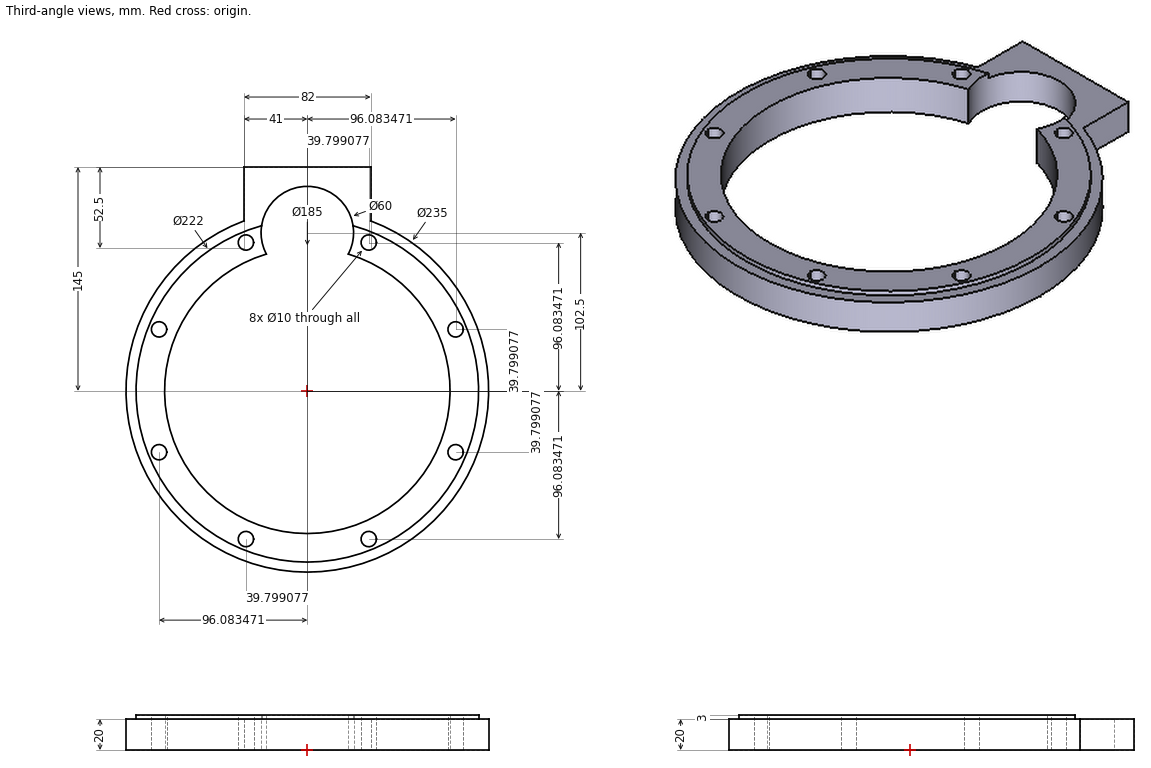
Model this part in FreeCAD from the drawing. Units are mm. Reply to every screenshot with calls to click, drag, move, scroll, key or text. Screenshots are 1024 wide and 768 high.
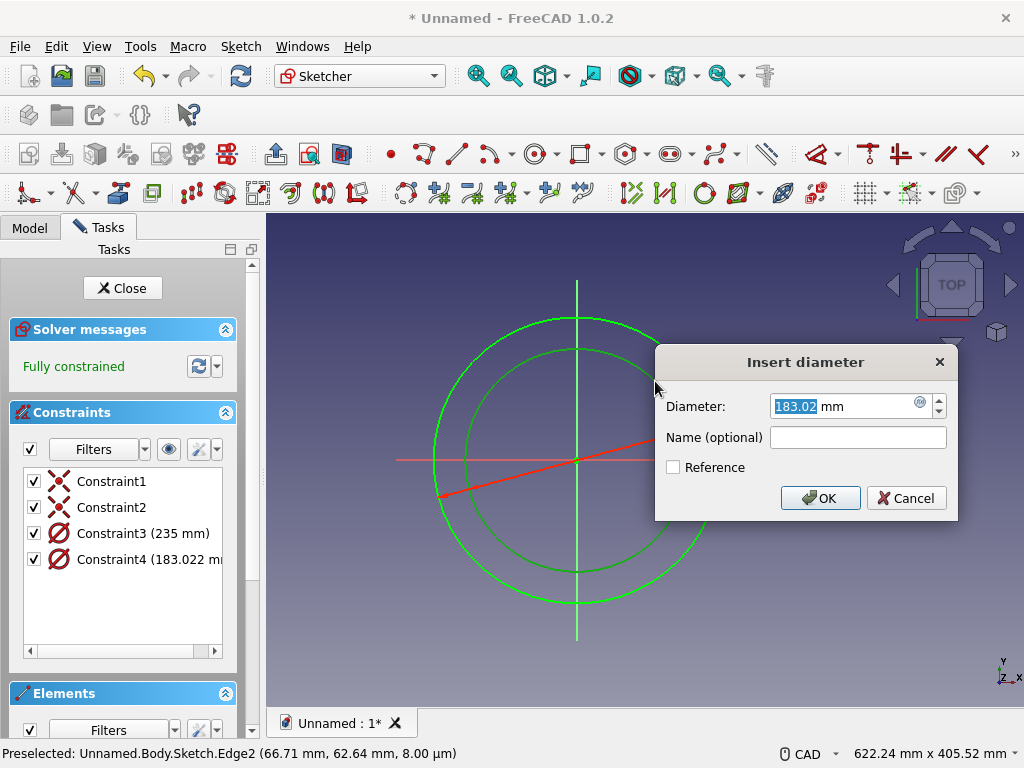
text(185)
key(Return)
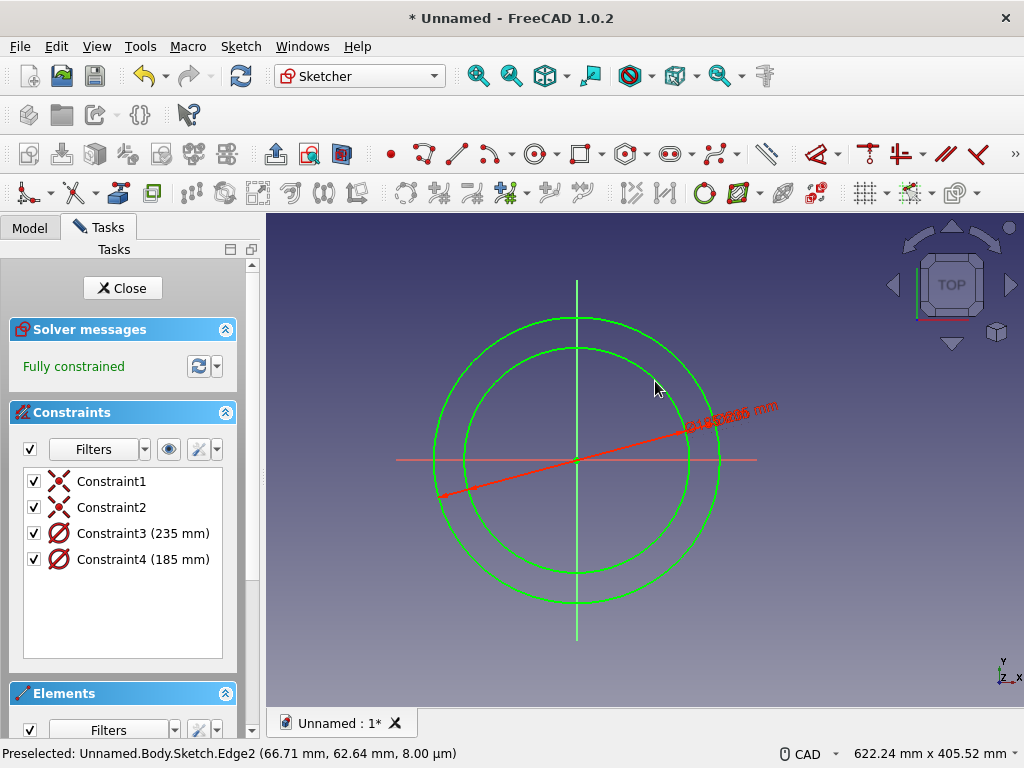
click(123, 288)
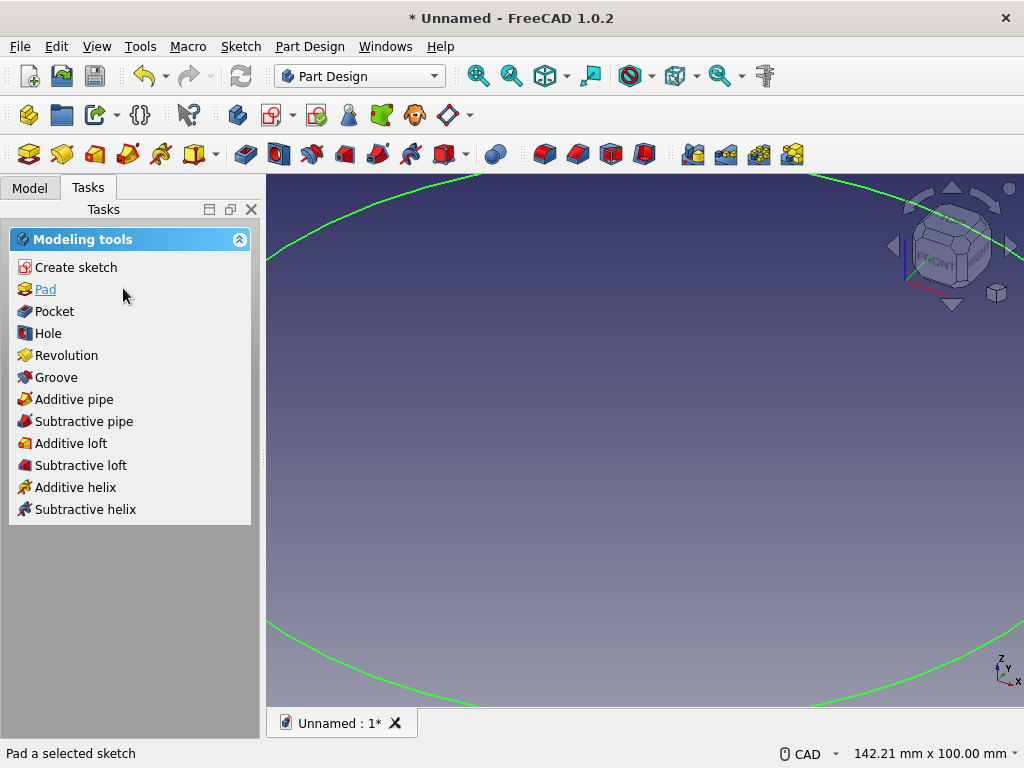
click(29, 154)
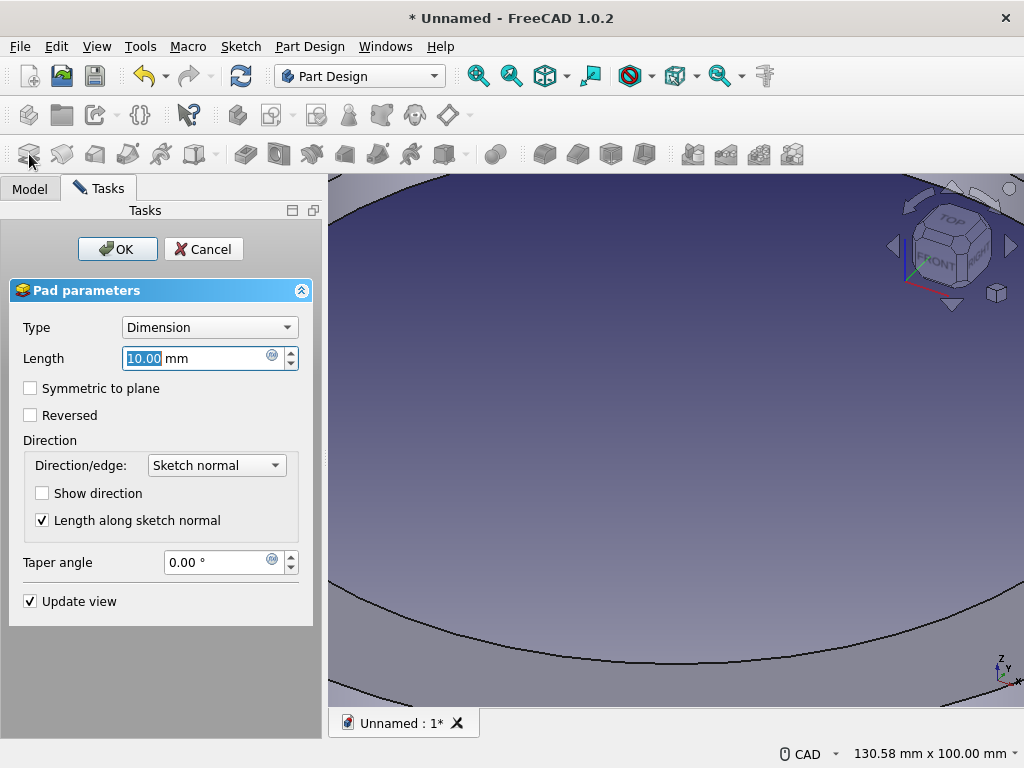
text(20)
key(Tab)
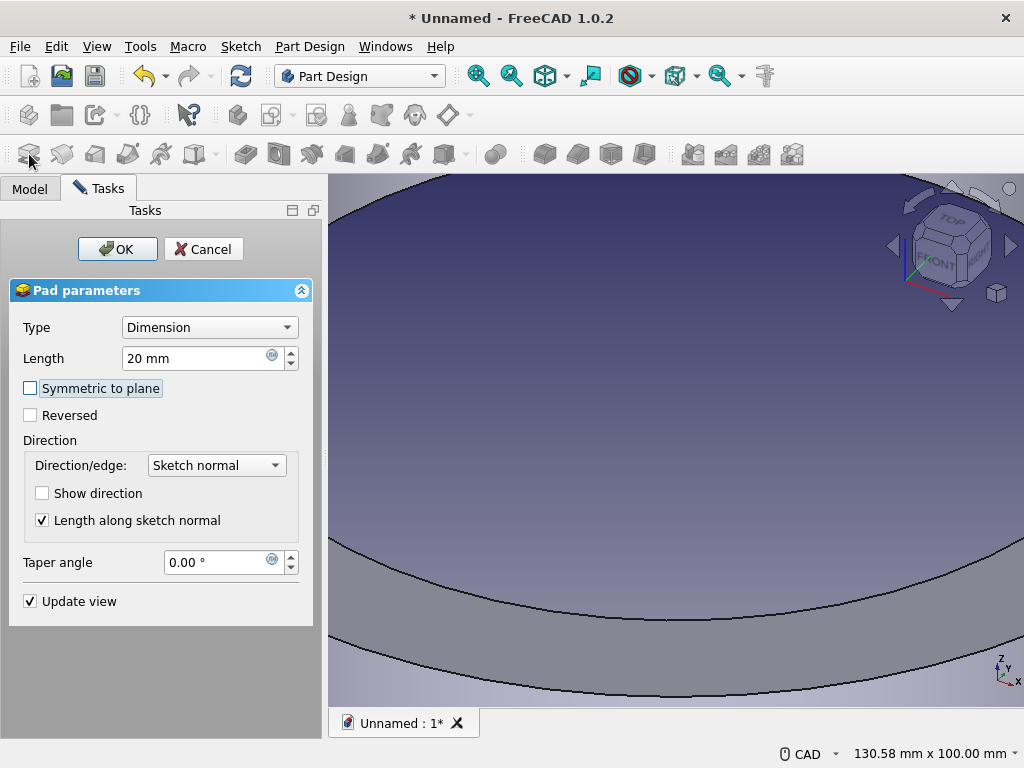
click(118, 249)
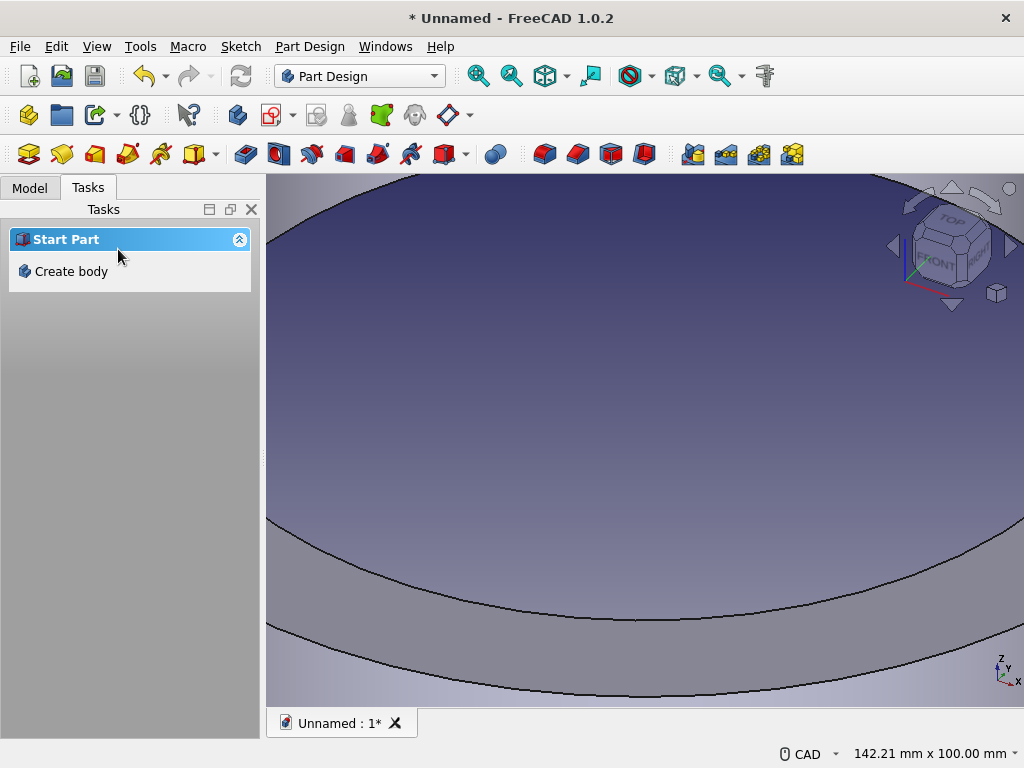
click(479, 76)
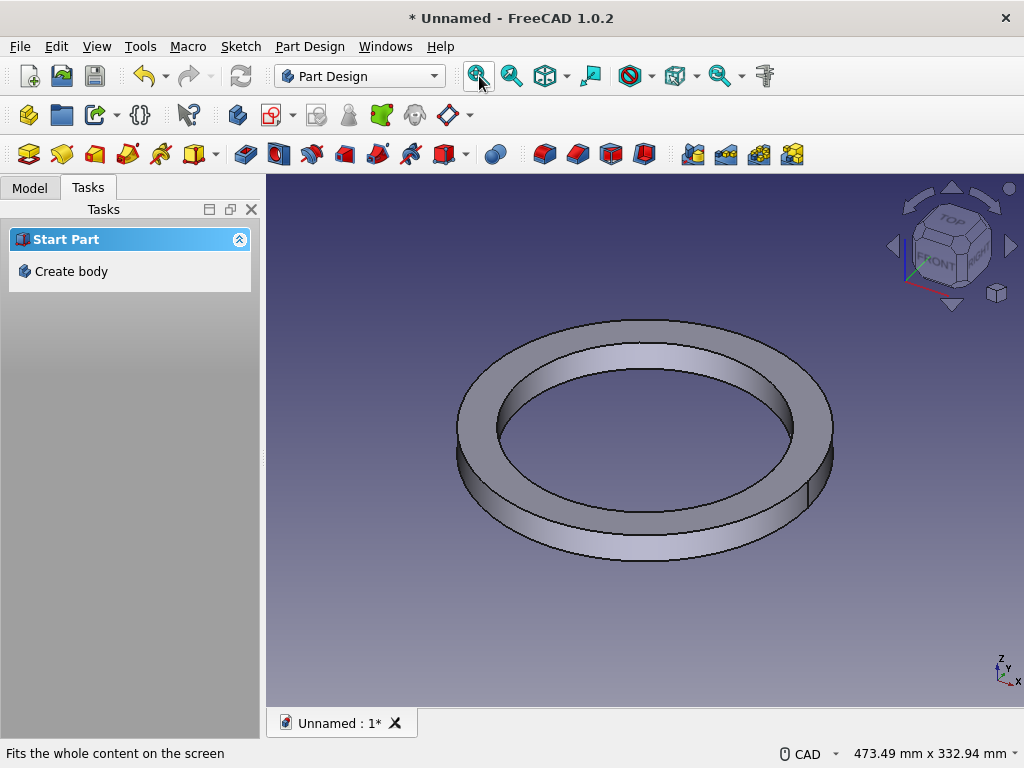
click(758, 499)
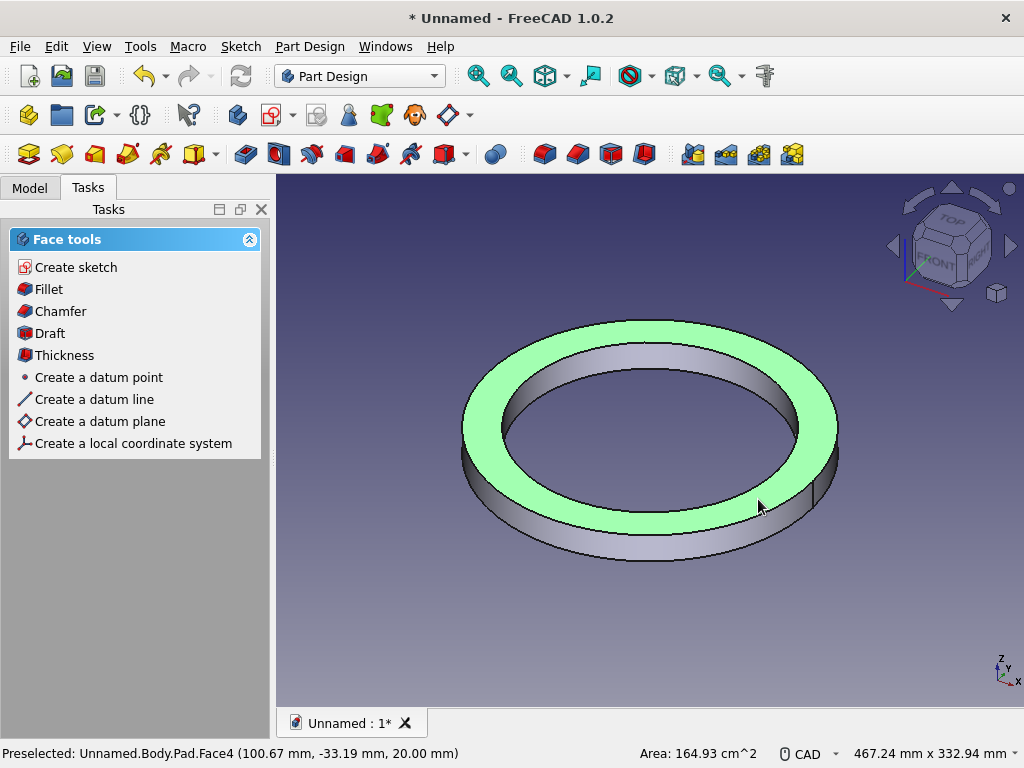
click(270, 116)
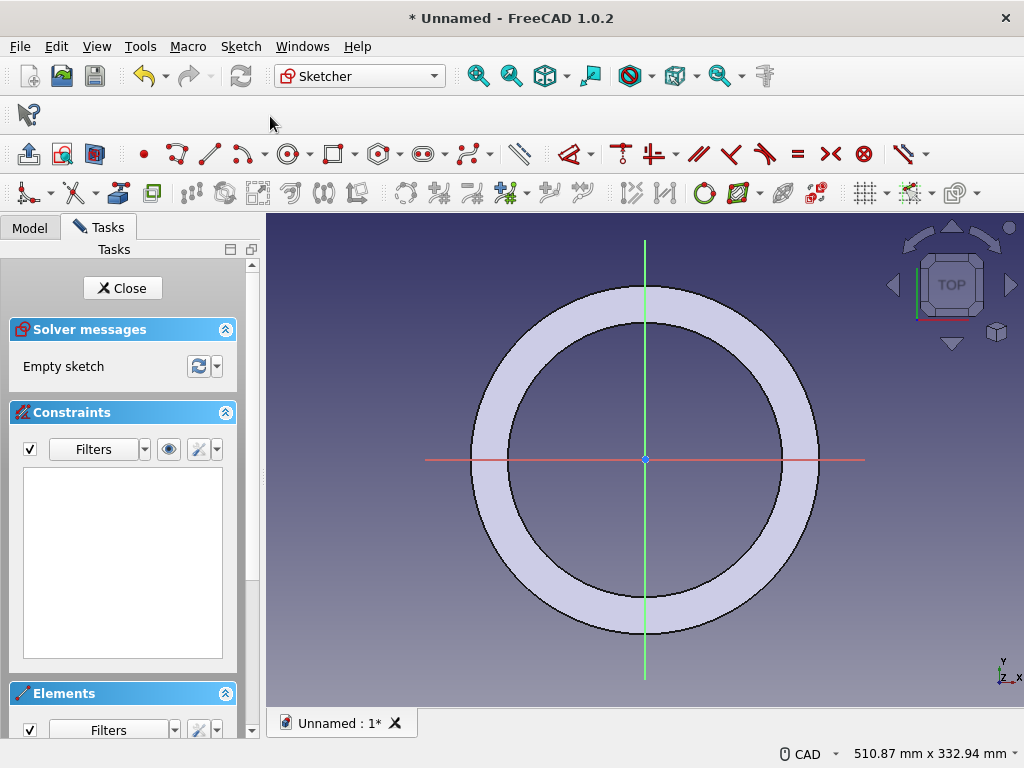
scroll(294, 679, down, 1)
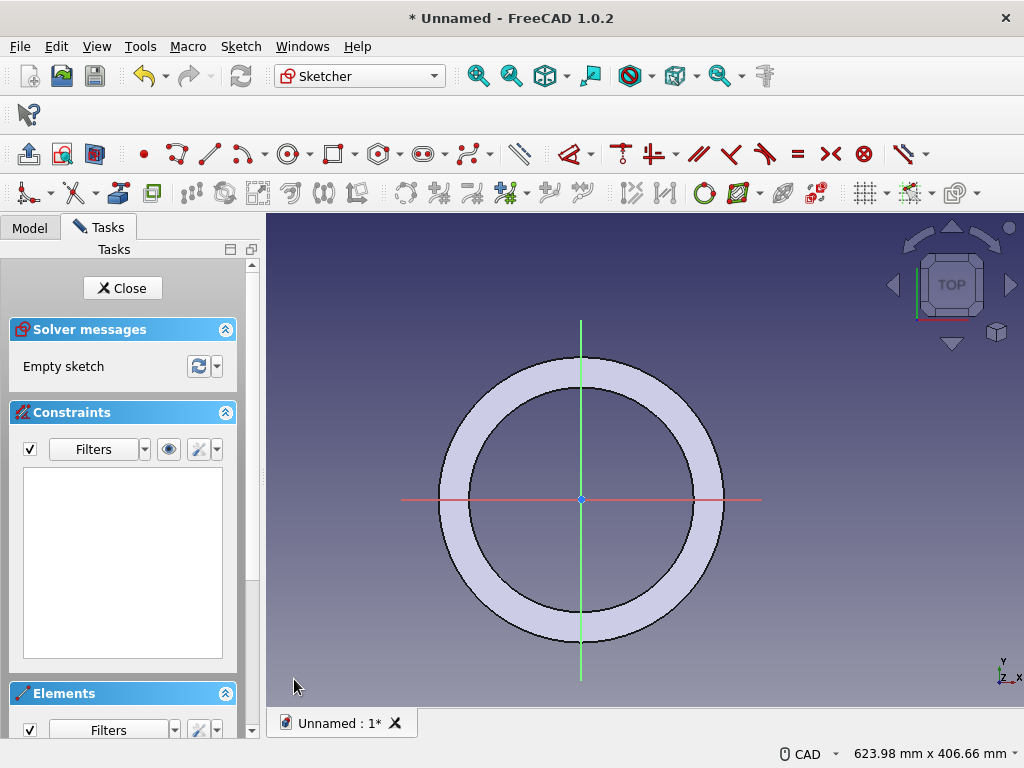
scroll(587, 353, up, 3)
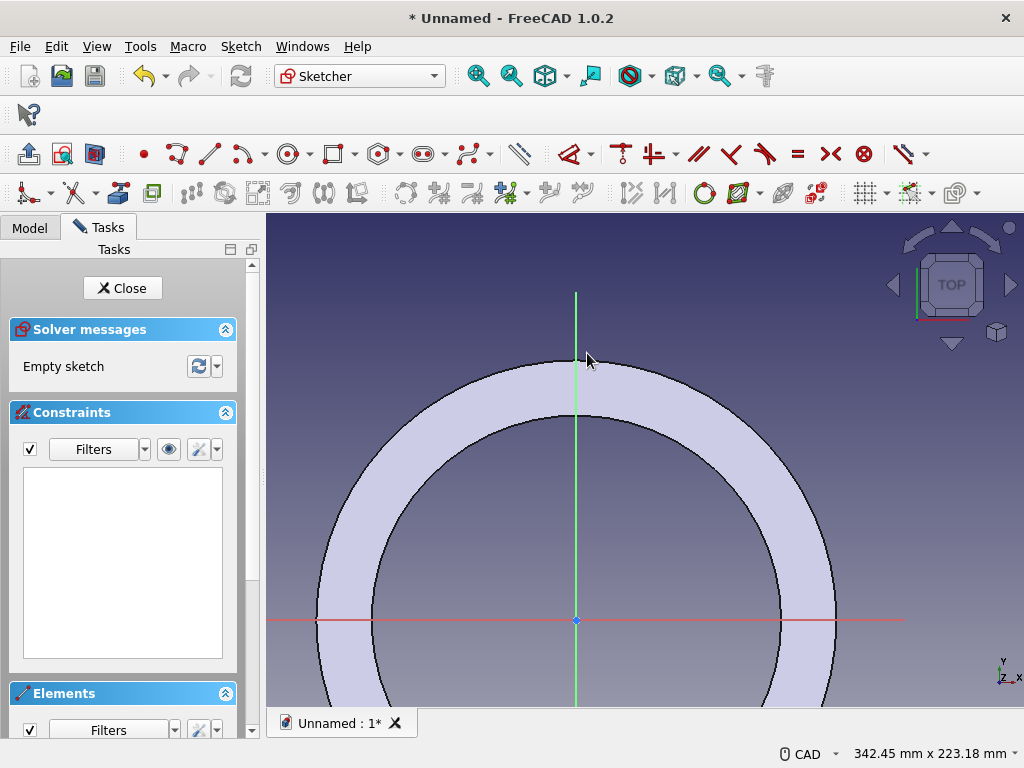
click(332, 154)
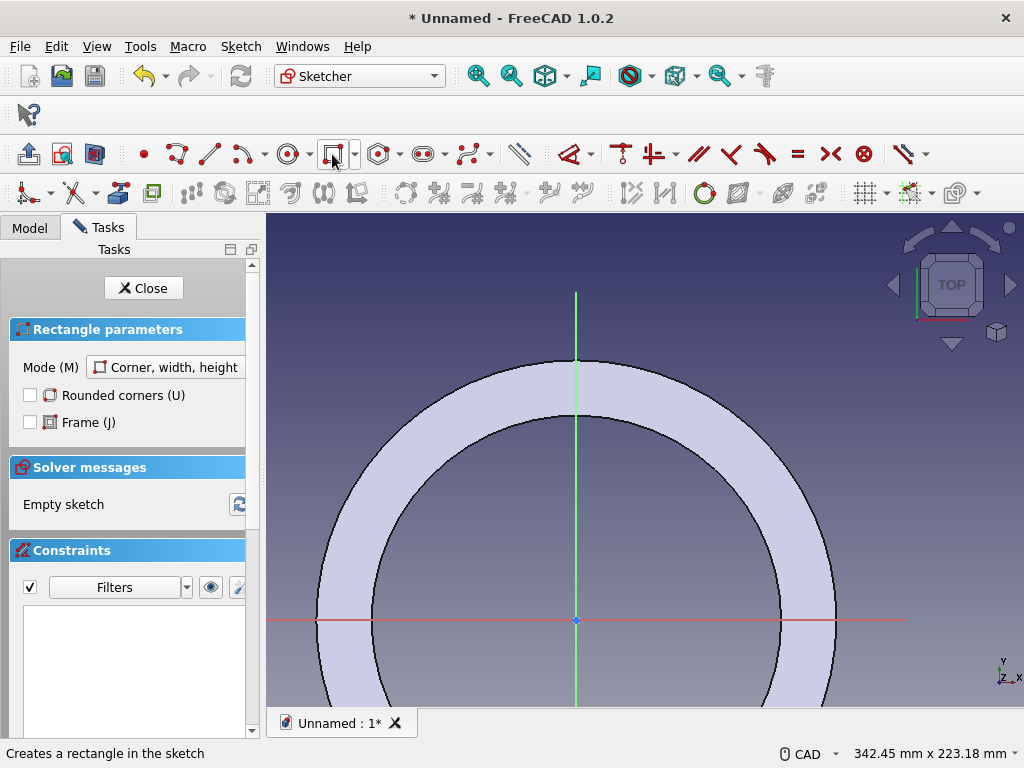
click(486, 299)
click(667, 416)
key(Escape)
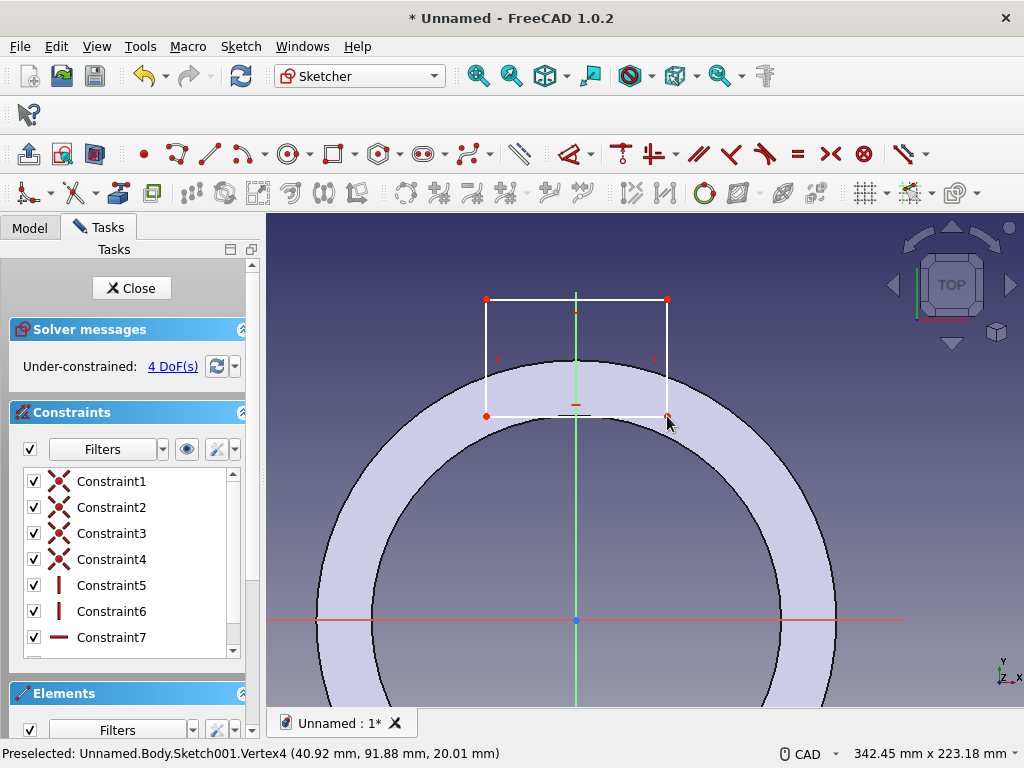
click(540, 417)